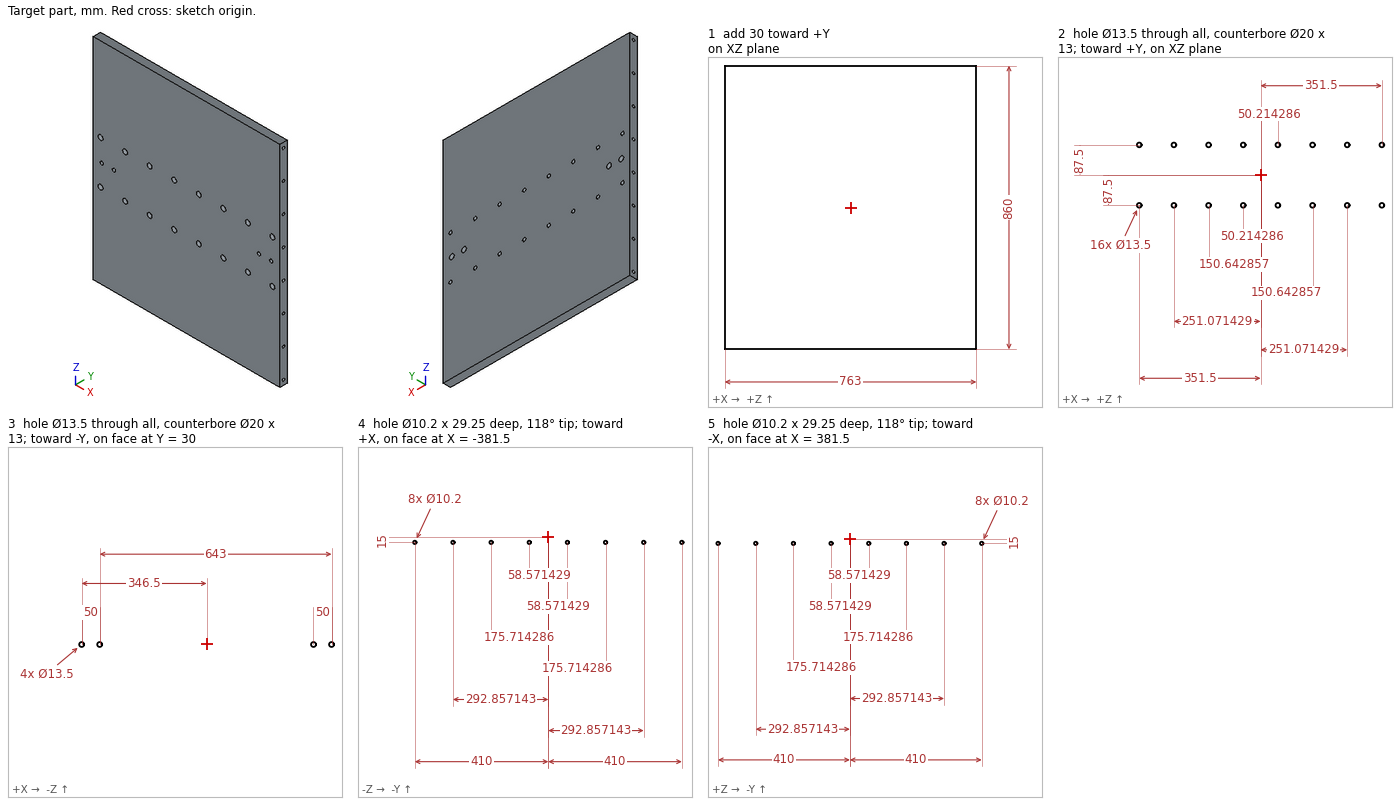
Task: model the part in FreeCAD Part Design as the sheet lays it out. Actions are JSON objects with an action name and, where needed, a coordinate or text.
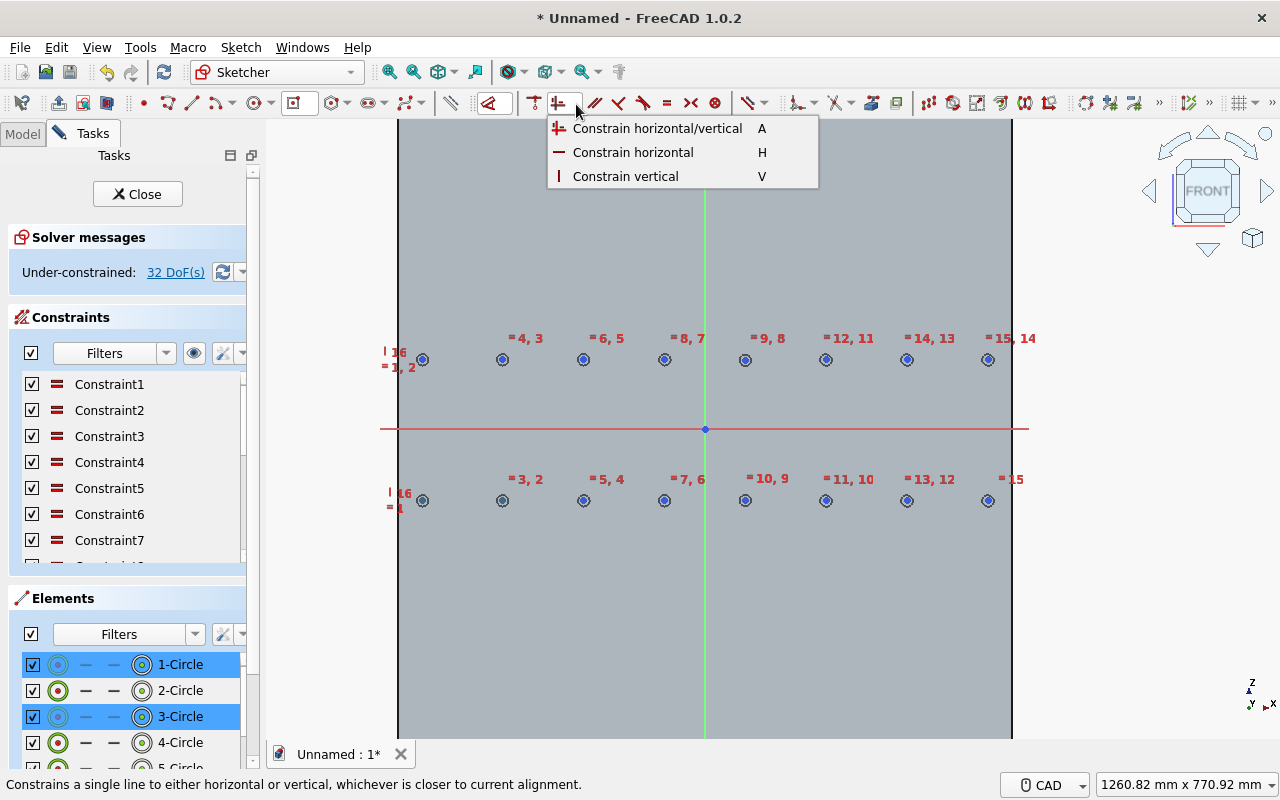
{"action": "left_click", "coordinate": [683, 152]}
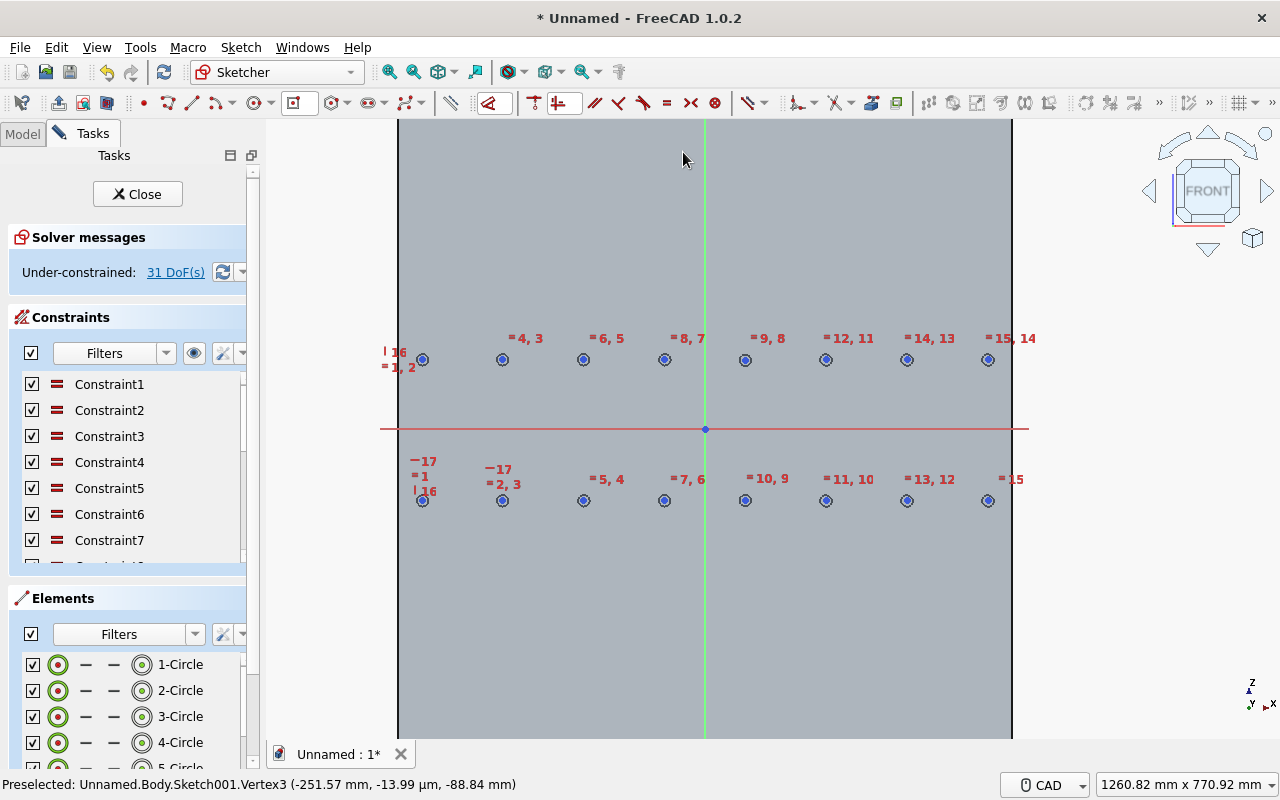
{"action": "left_click", "coordinate": [503, 501]}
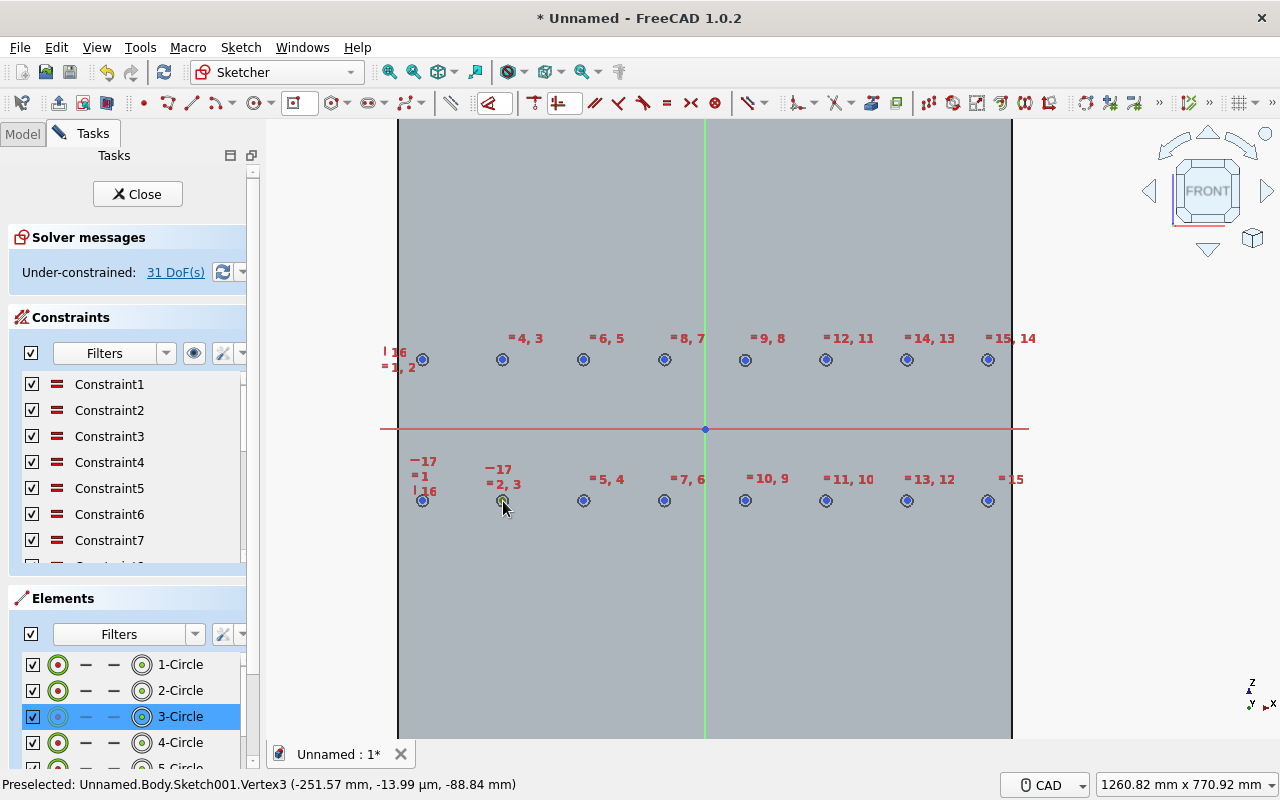
{"action": "left_click", "coordinate": [503, 360]}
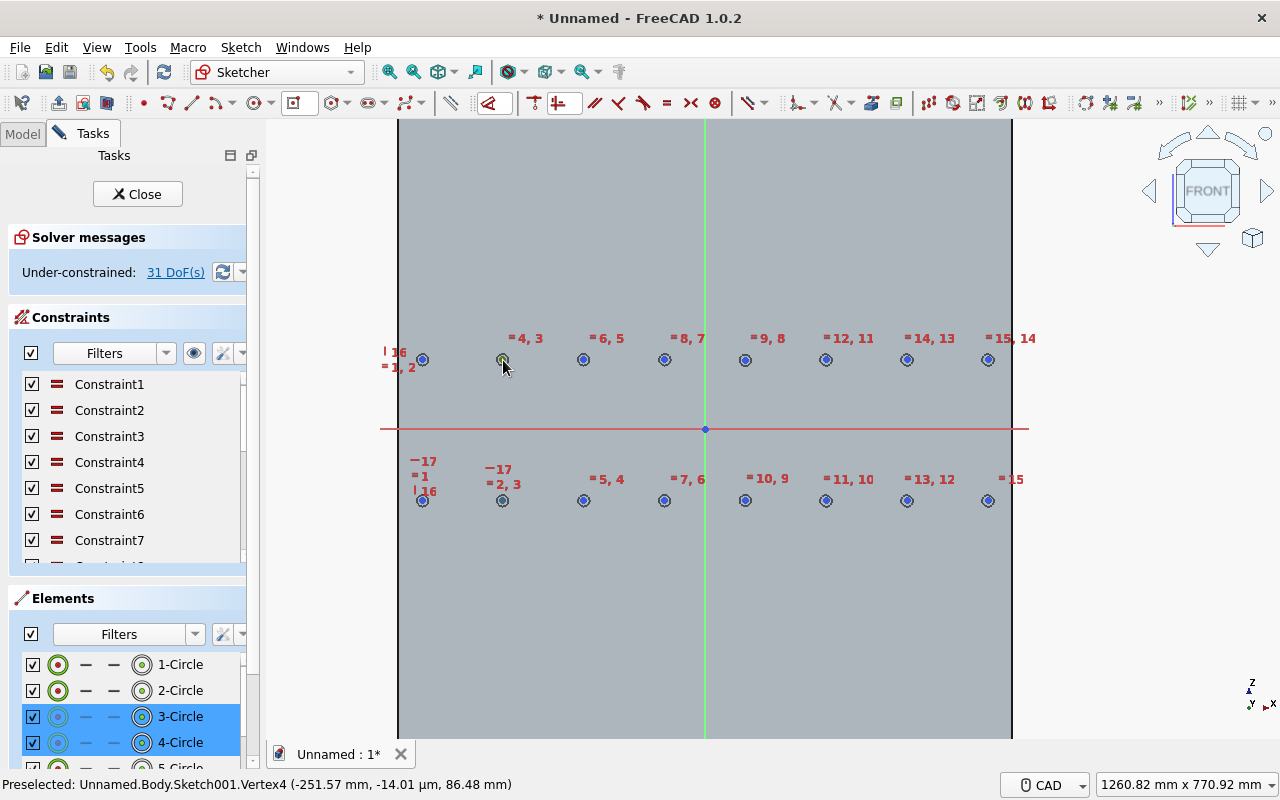
{"action": "left_click", "coordinate": [576, 104]}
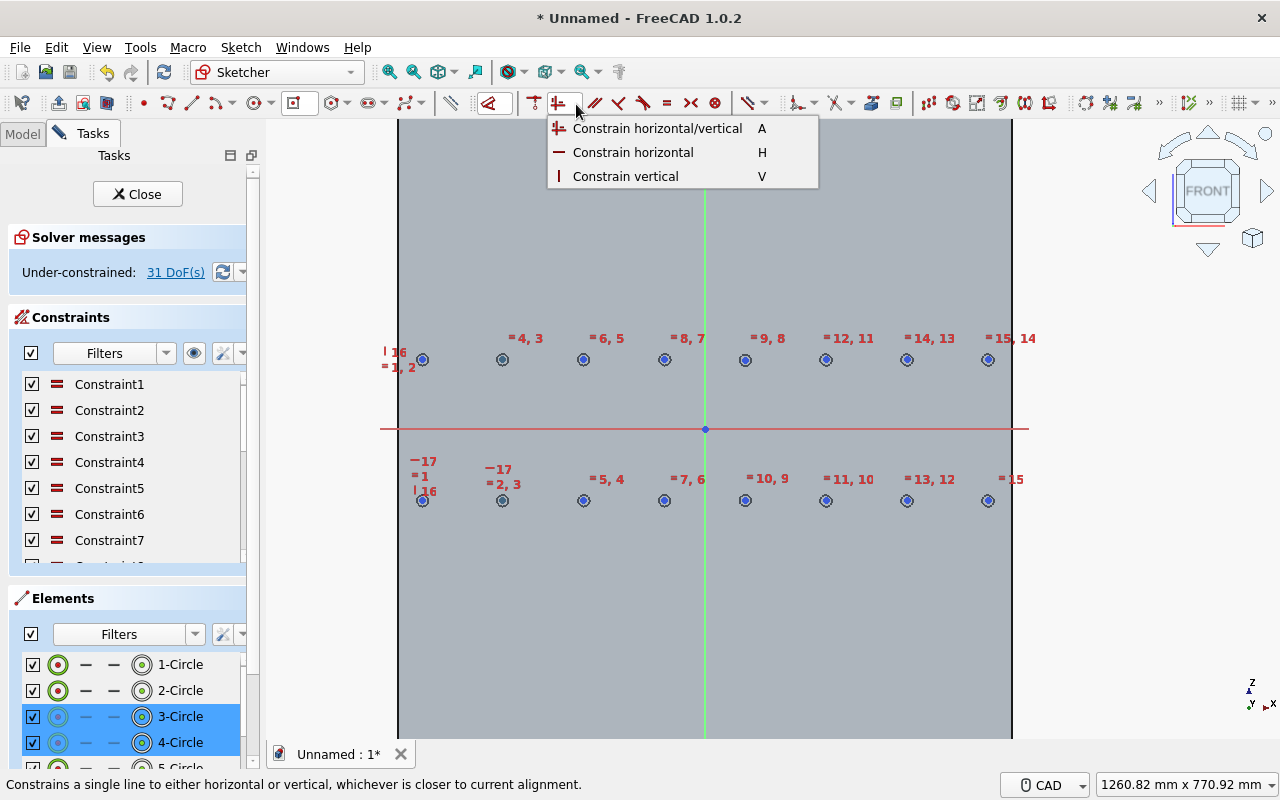
{"action": "left_click", "coordinate": [683, 176]}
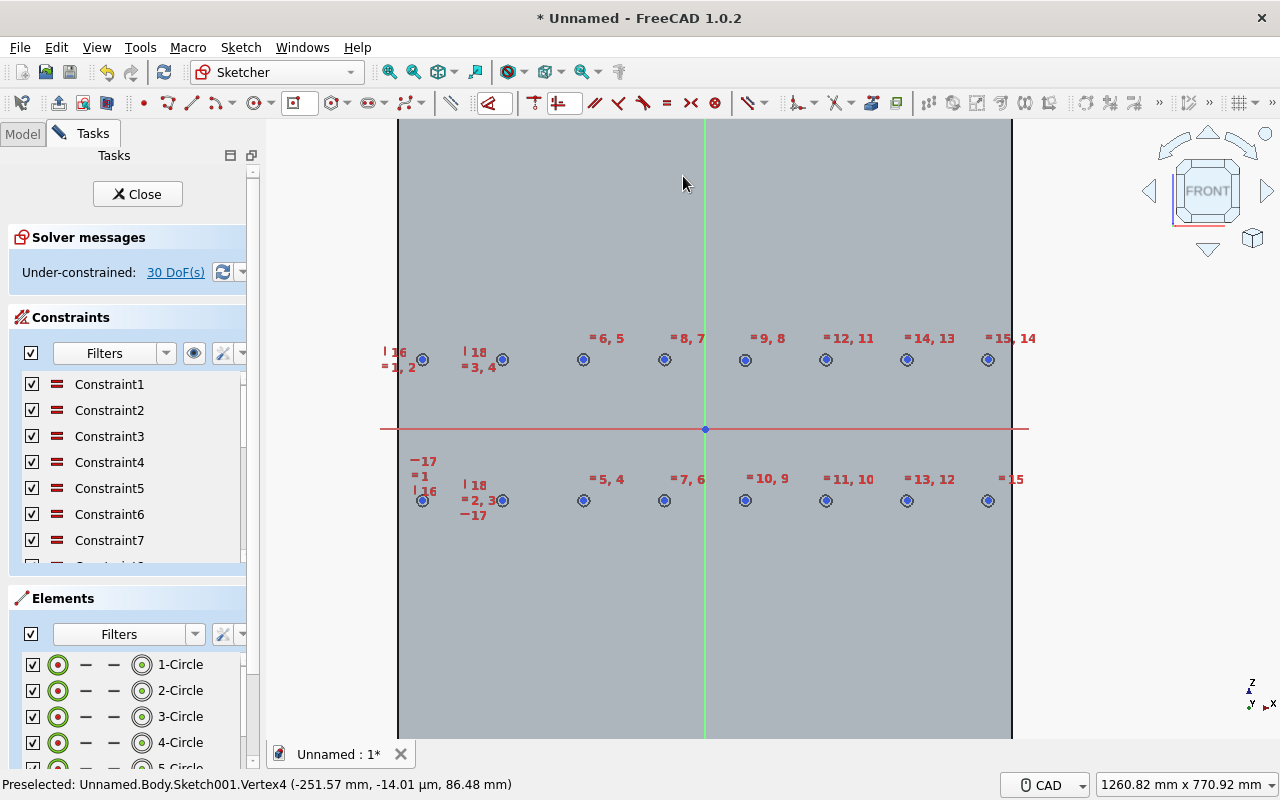
{"action": "left_click", "coordinate": [423, 360]}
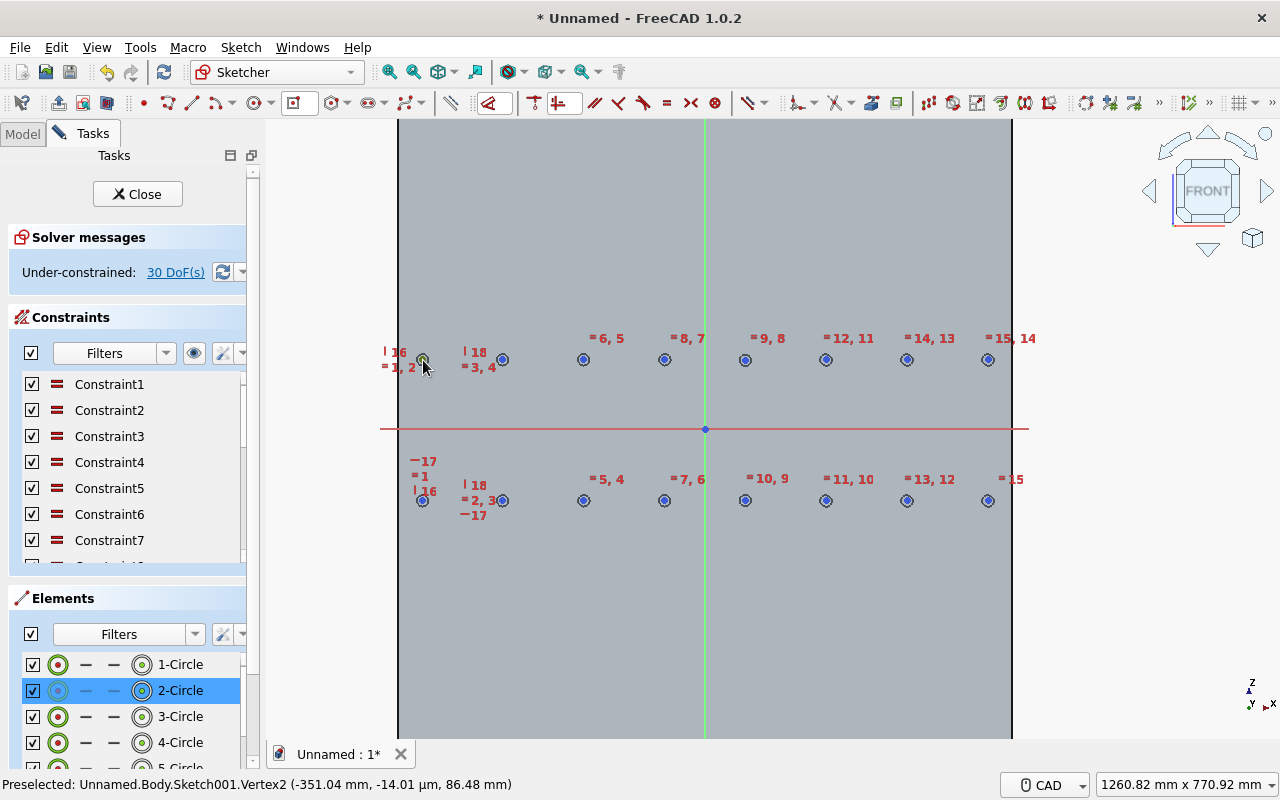
{"action": "left_click", "coordinate": [503, 360]}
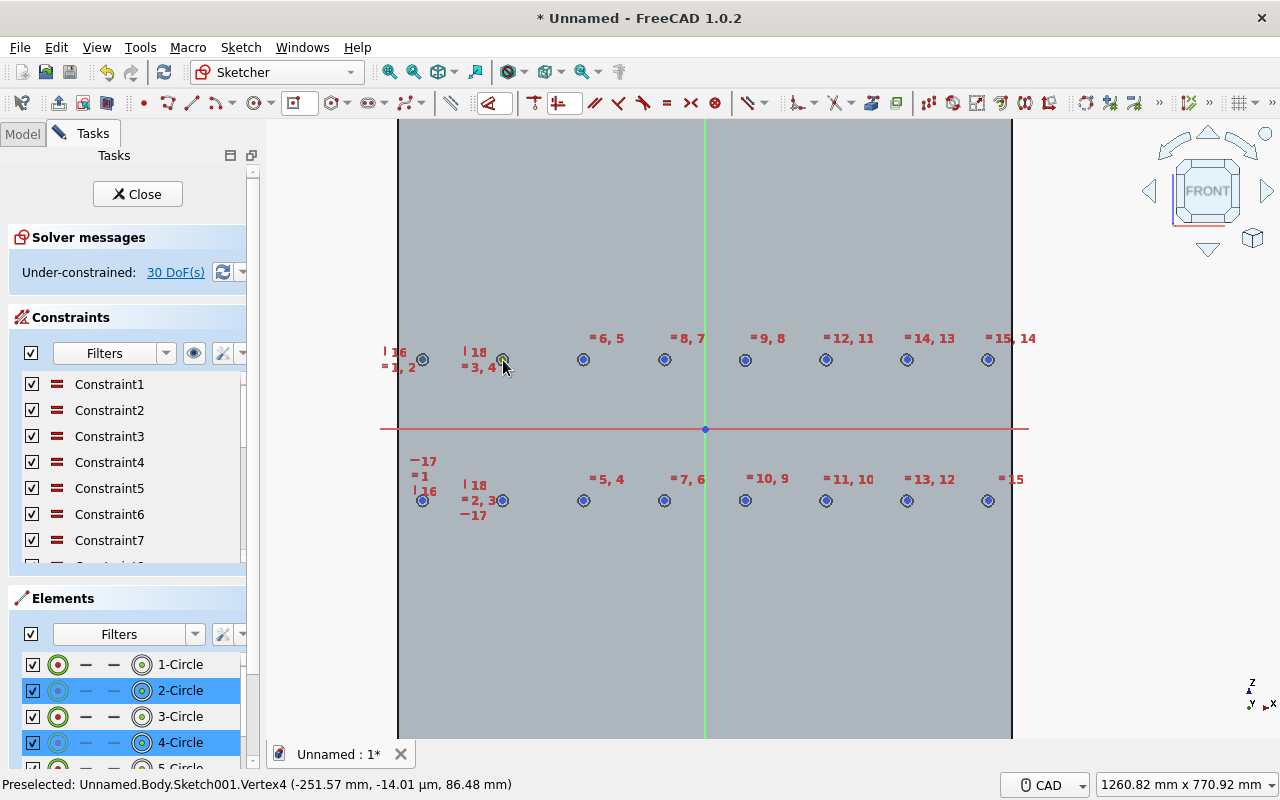
{"action": "left_click", "coordinate": [576, 104]}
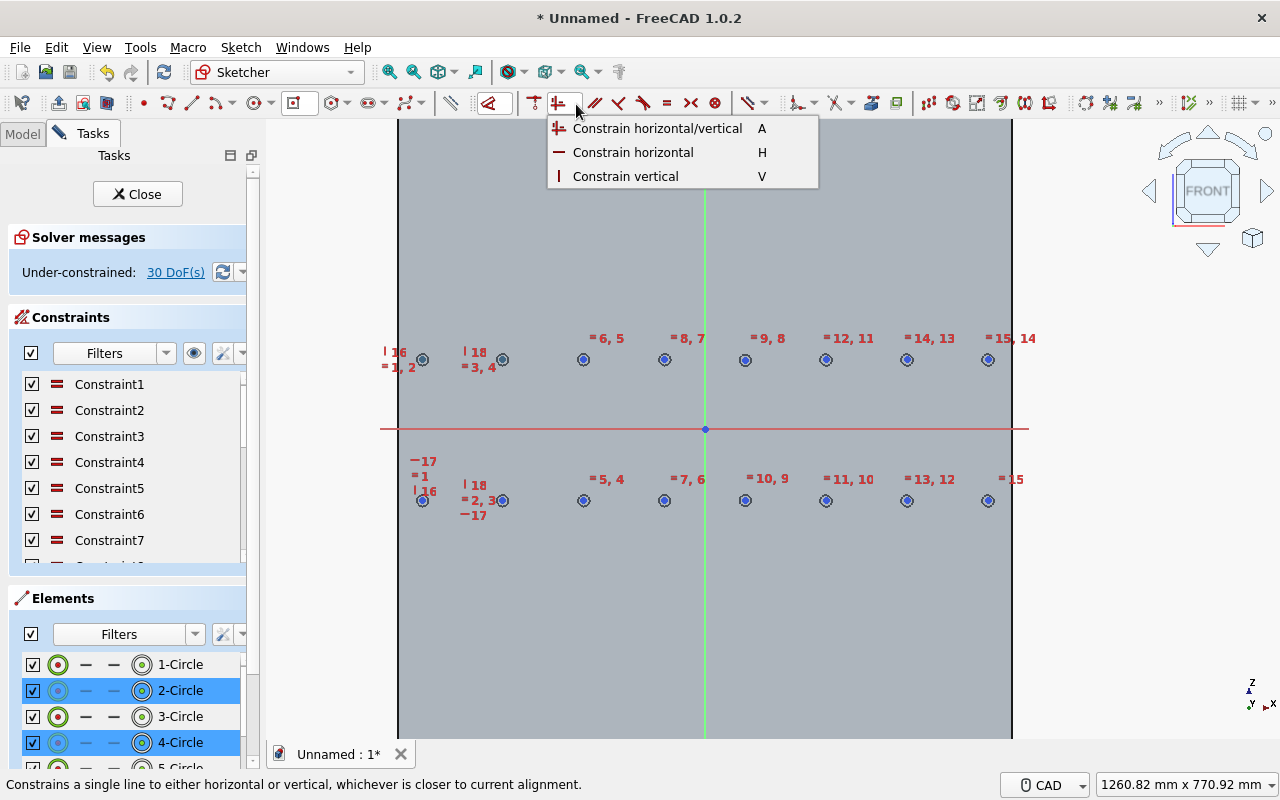
{"action": "left_click", "coordinate": [683, 152]}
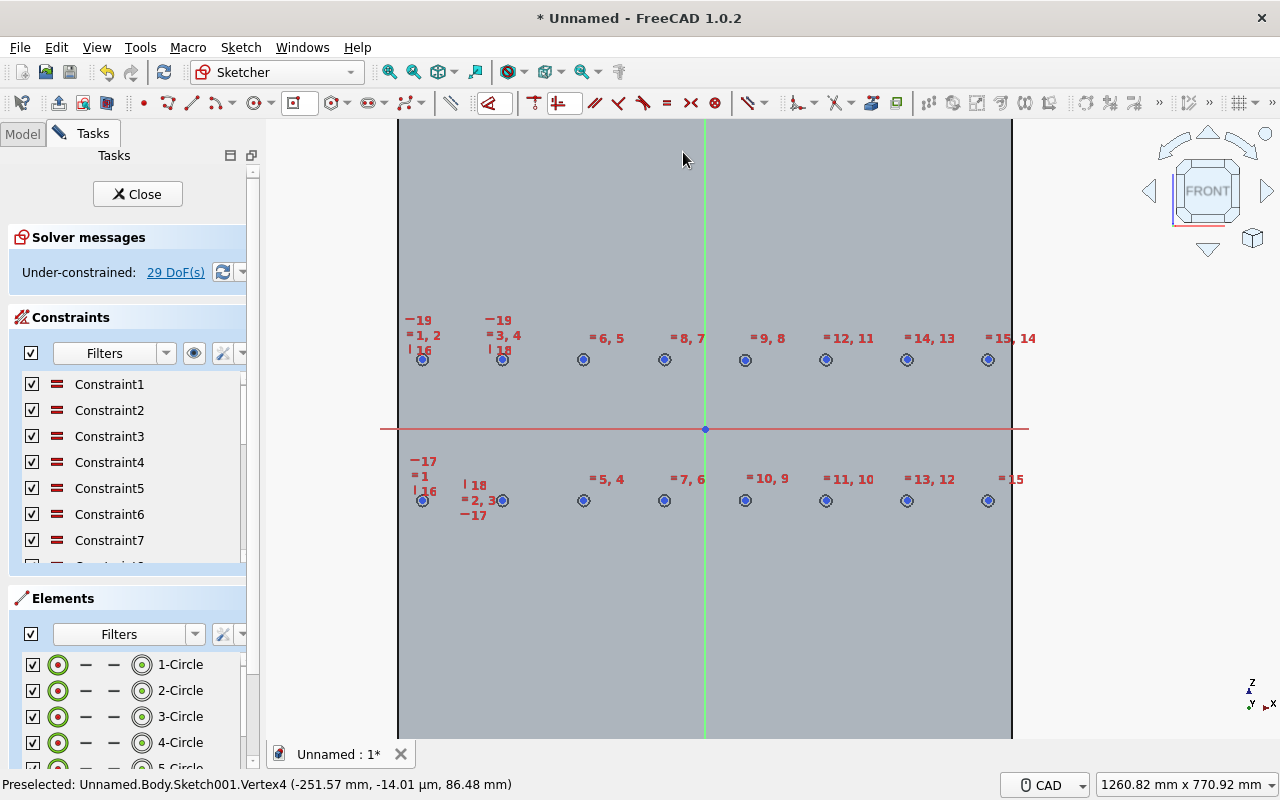
{"action": "left_click", "coordinate": [503, 501]}